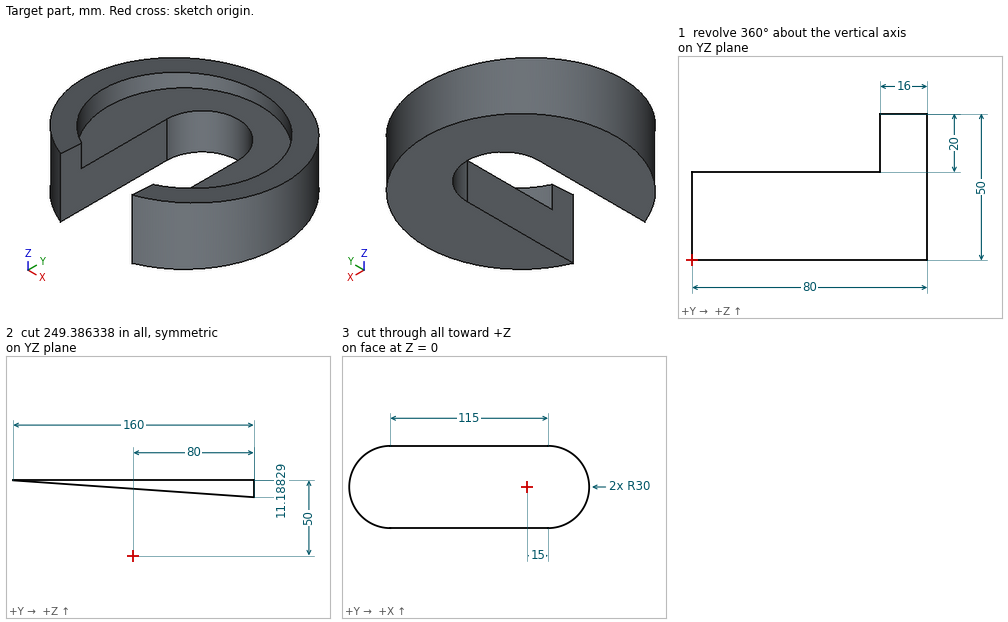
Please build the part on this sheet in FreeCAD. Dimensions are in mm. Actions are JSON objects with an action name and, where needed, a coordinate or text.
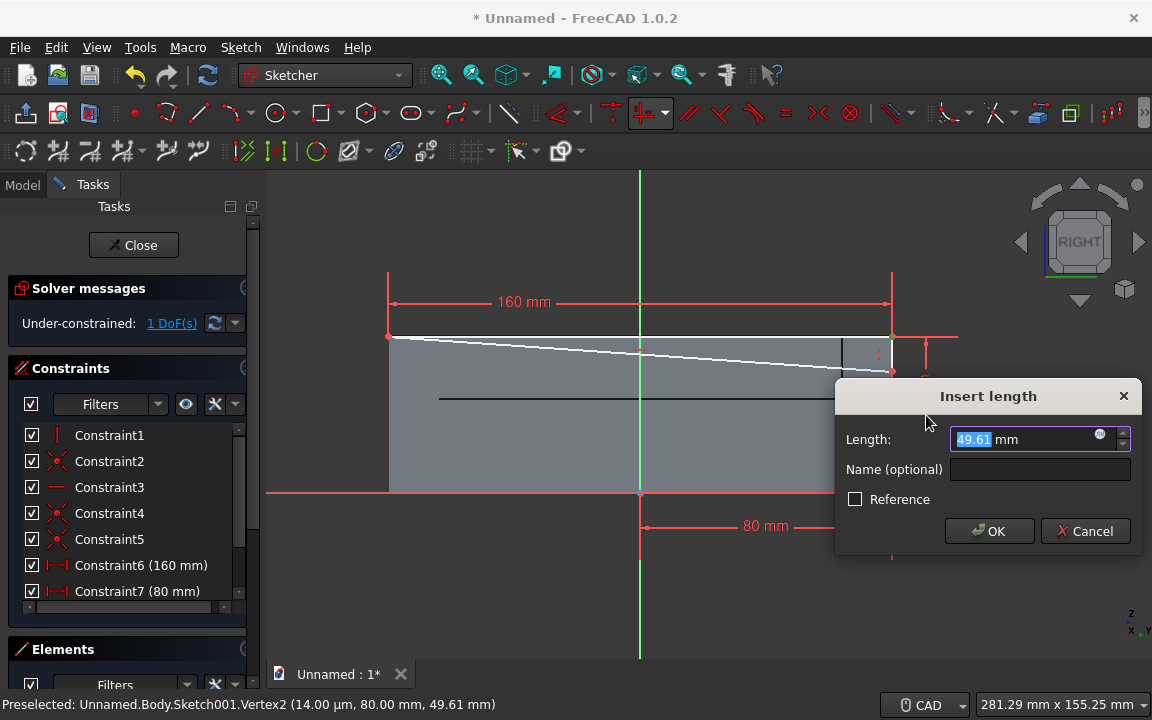
{"action": "type", "text": "50"}
{"action": "key", "text": "Return"}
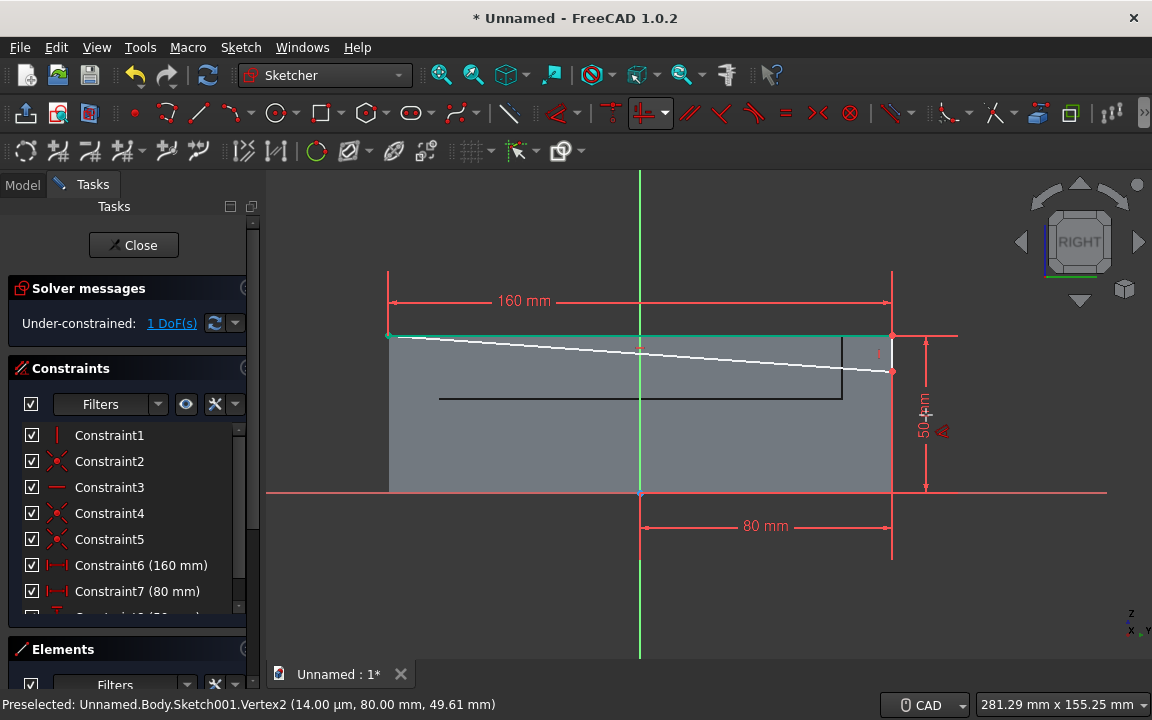
{"action": "scroll", "coordinate": [892, 361], "scroll_direction": "up", "scroll_amount": 2}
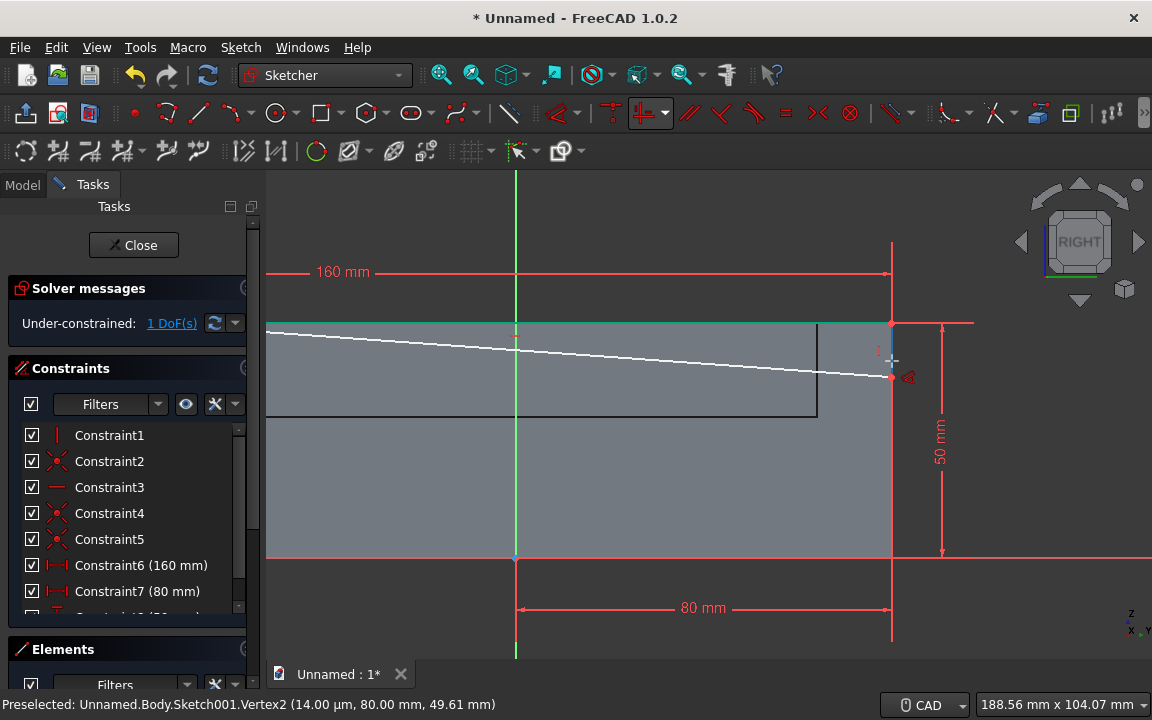
{"action": "left_click", "coordinate": [892, 361]}
{"action": "left_click", "coordinate": [926, 350]}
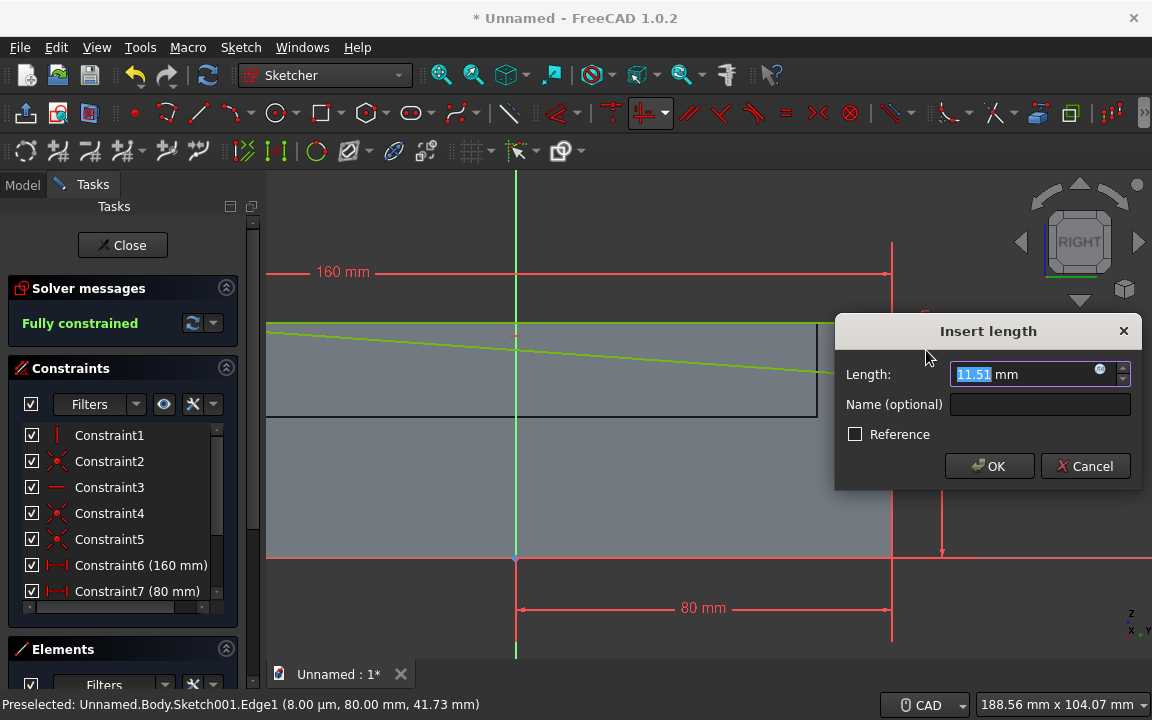
{"action": "type", "text": "11.18829"}
{"action": "key", "text": "Return"}
{"action": "key", "text": "Escape"}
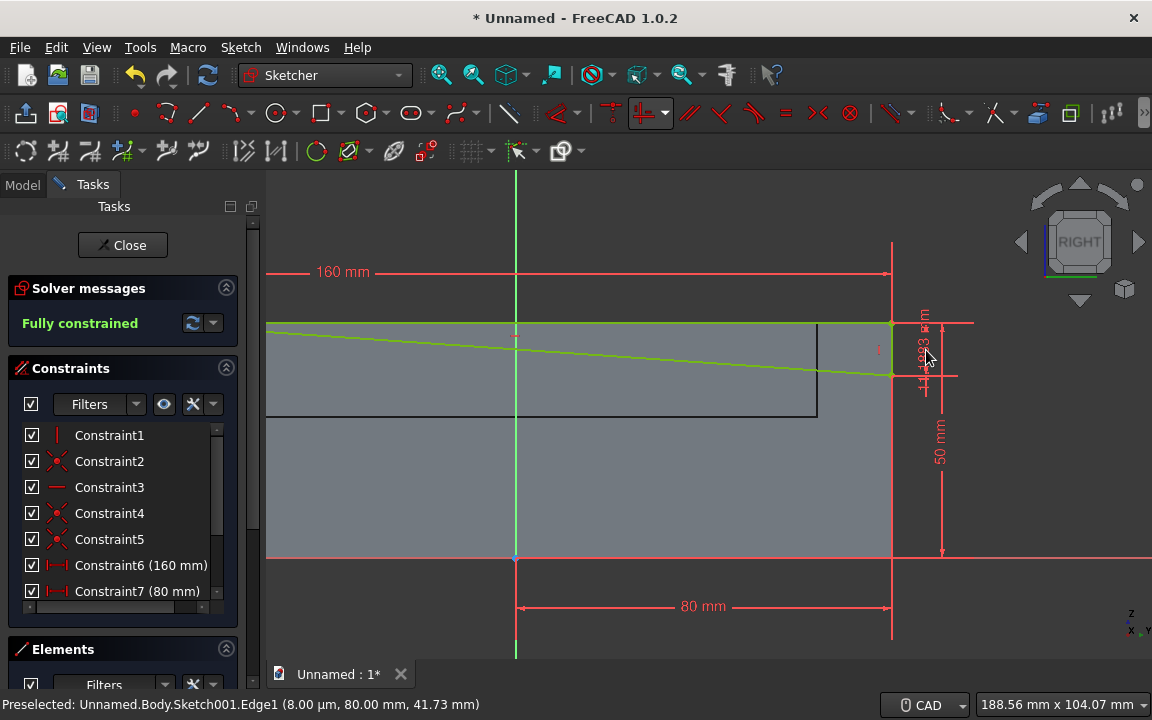
{"action": "left_click", "coordinate": [123, 245]}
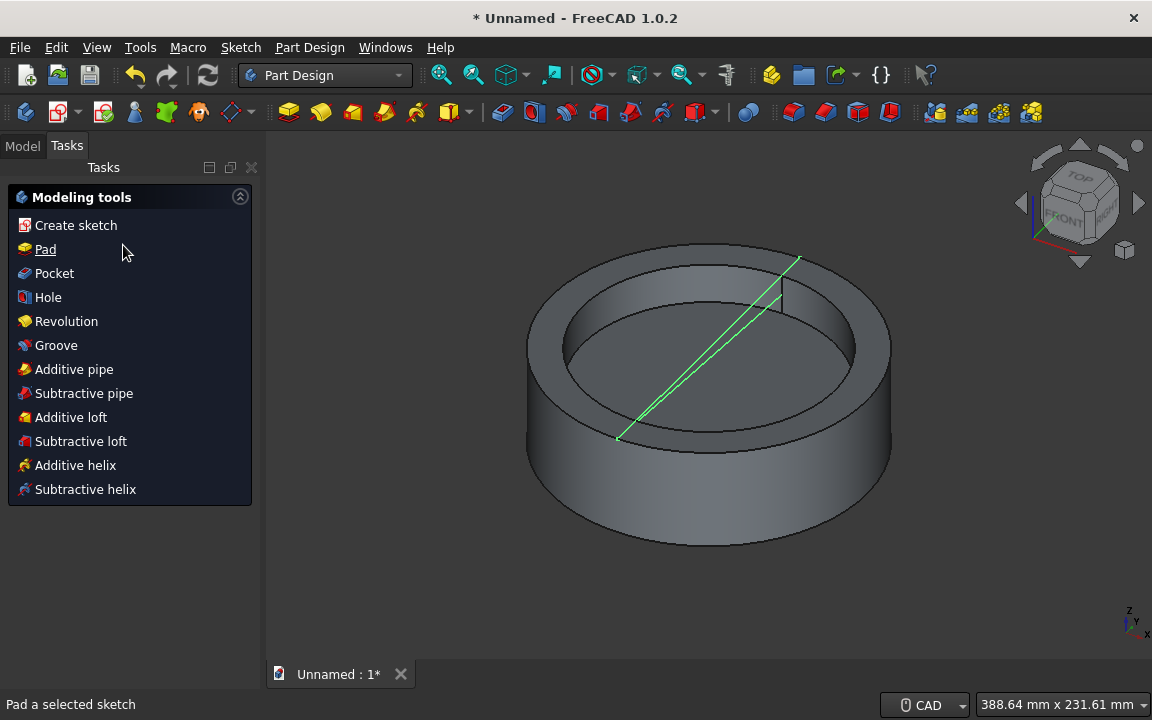
{"action": "left_click", "coordinate": [504, 112]}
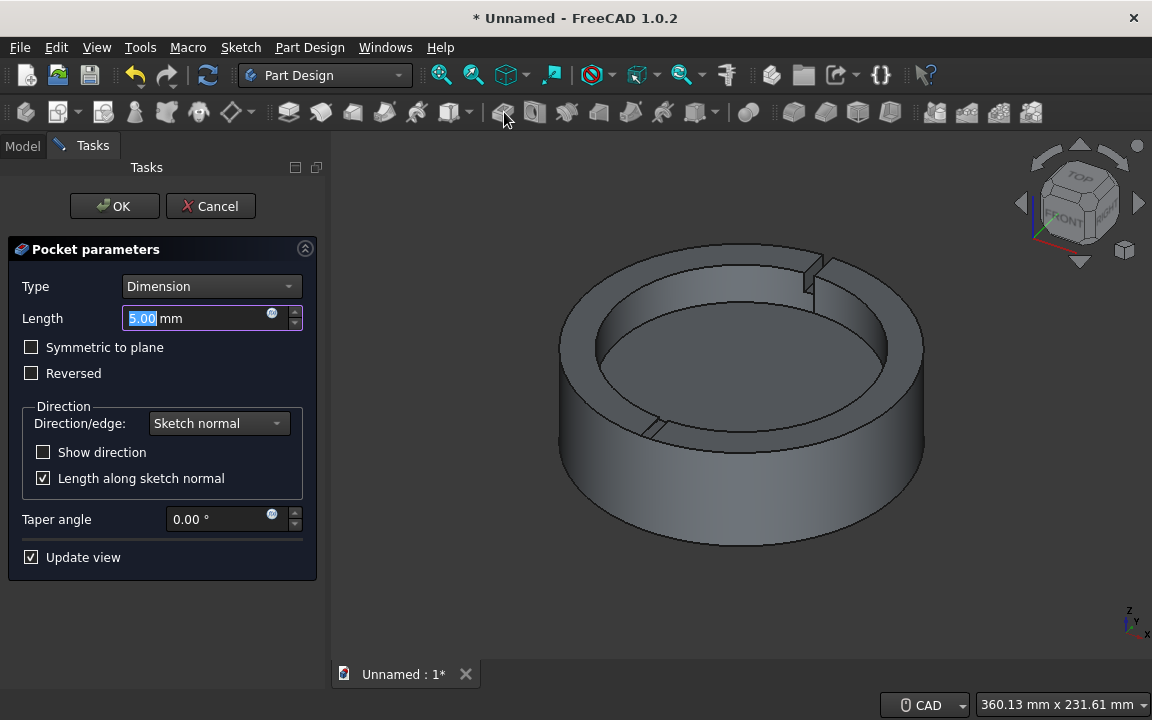
{"action": "type", "text": "249.386338"}
{"action": "key", "text": "Tab"}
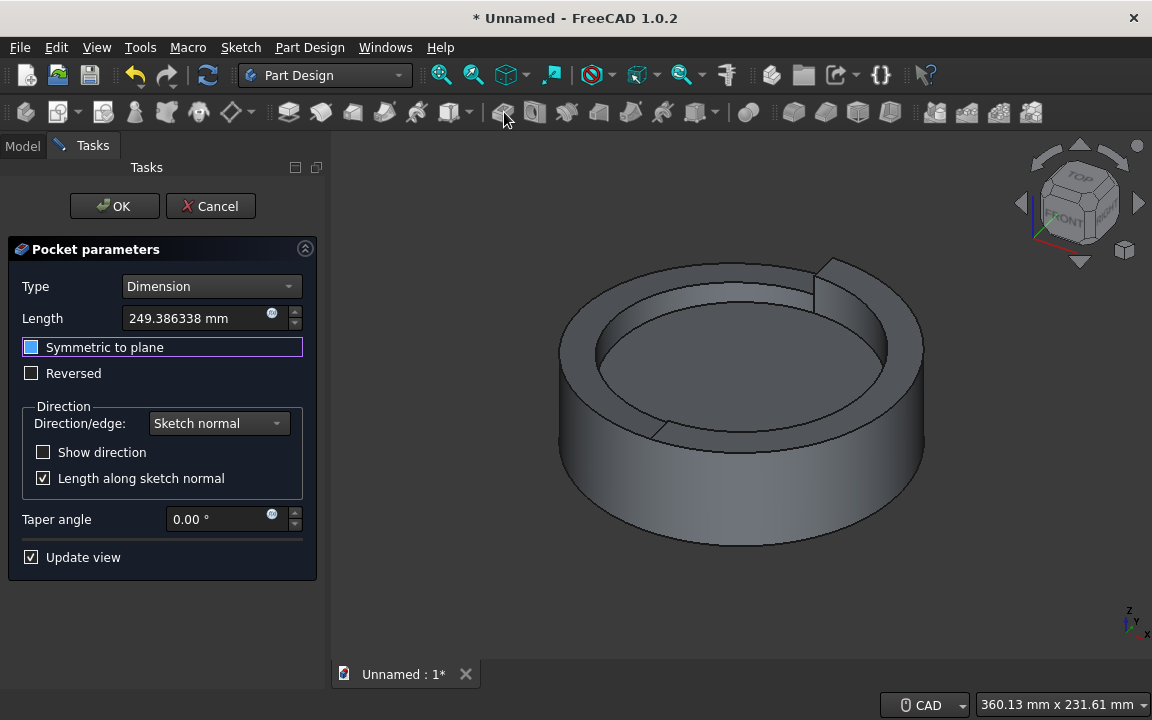
{"action": "left_click", "coordinate": [30, 347]}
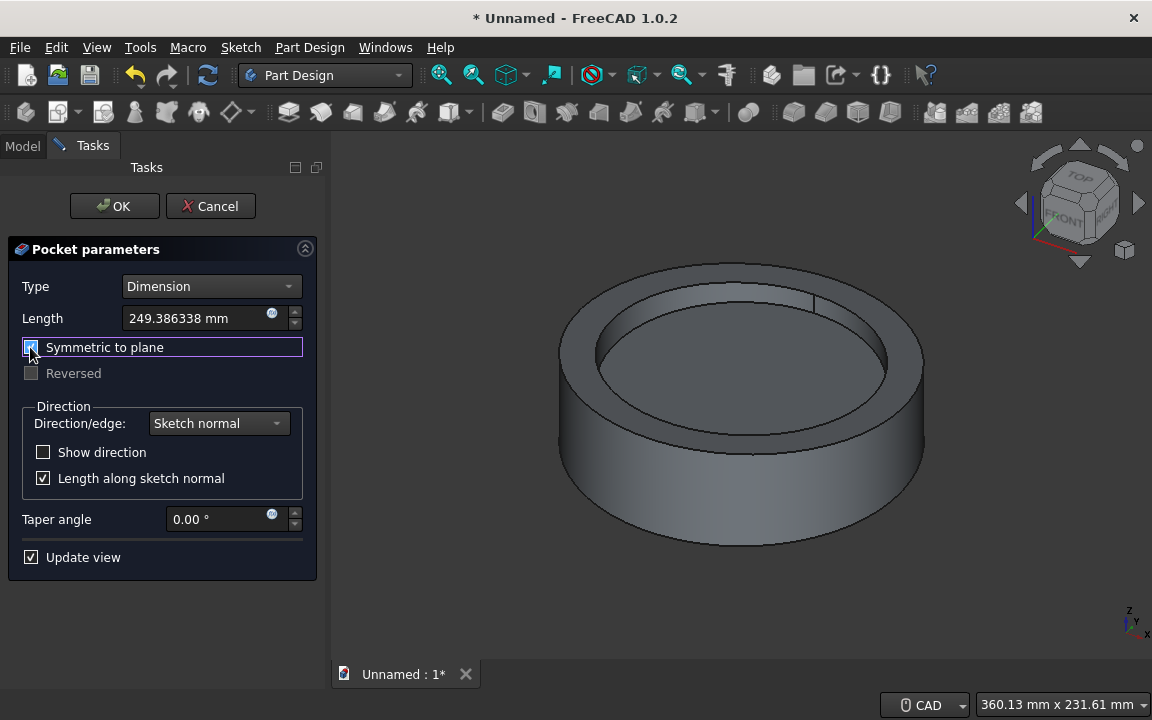
{"action": "left_click", "coordinate": [115, 206]}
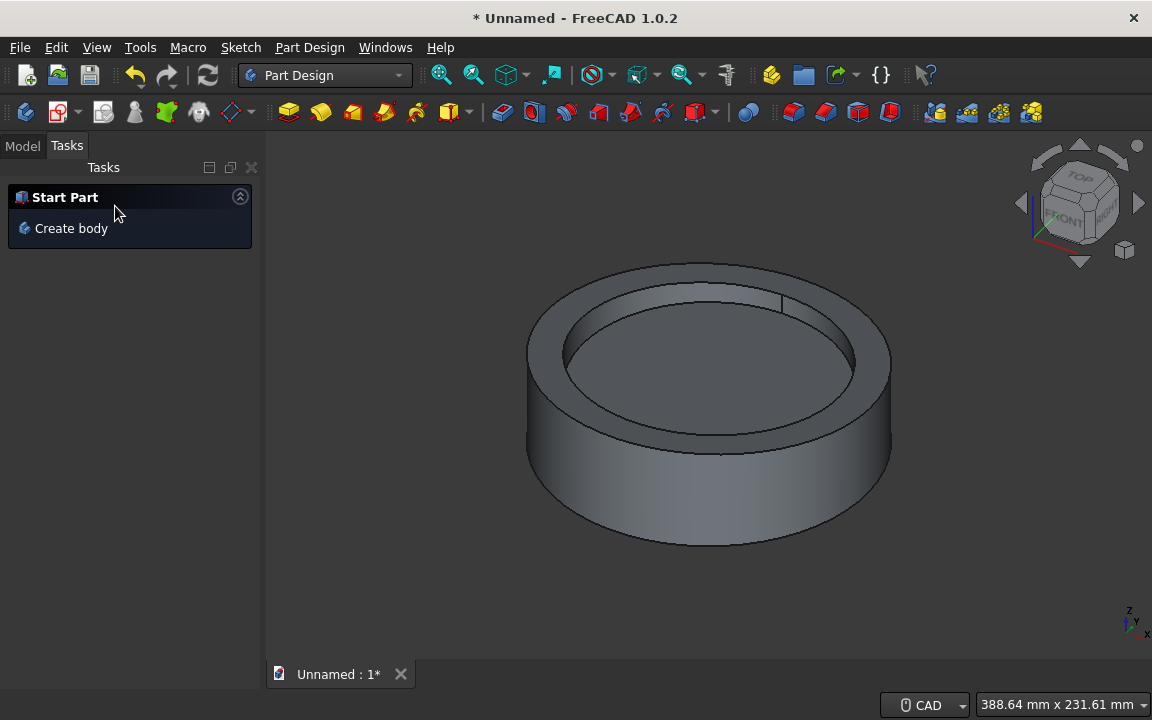
{"action": "key", "text": "5"}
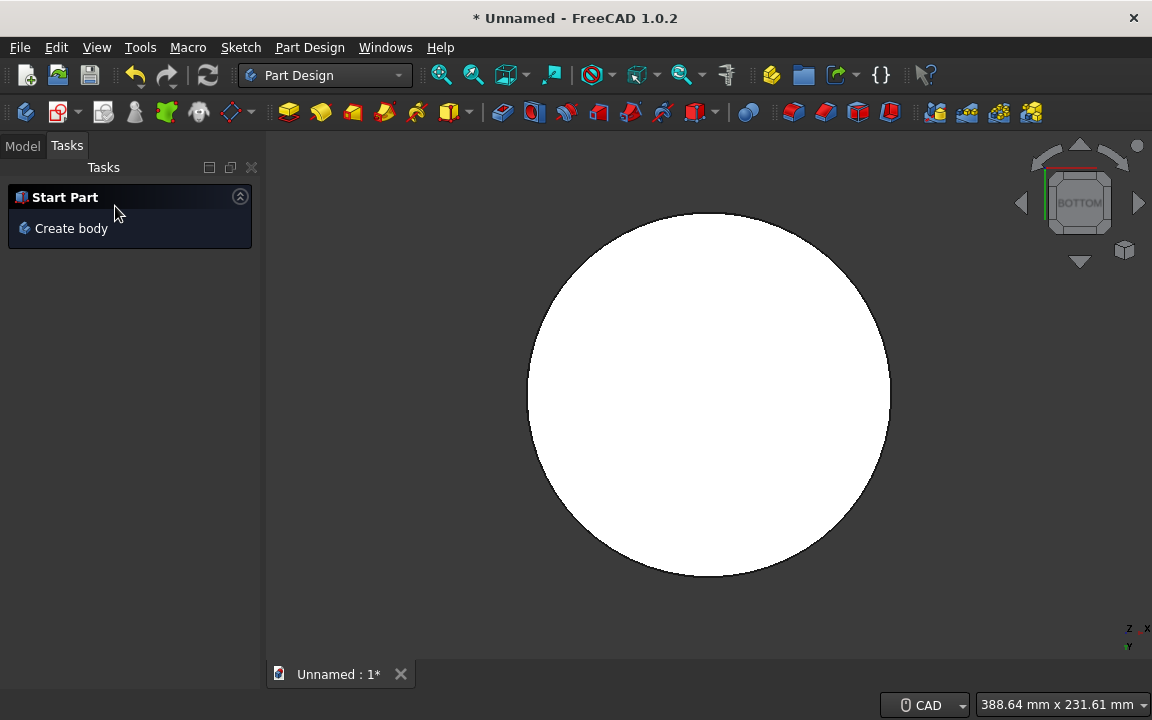
{"action": "left_click", "coordinate": [709, 394]}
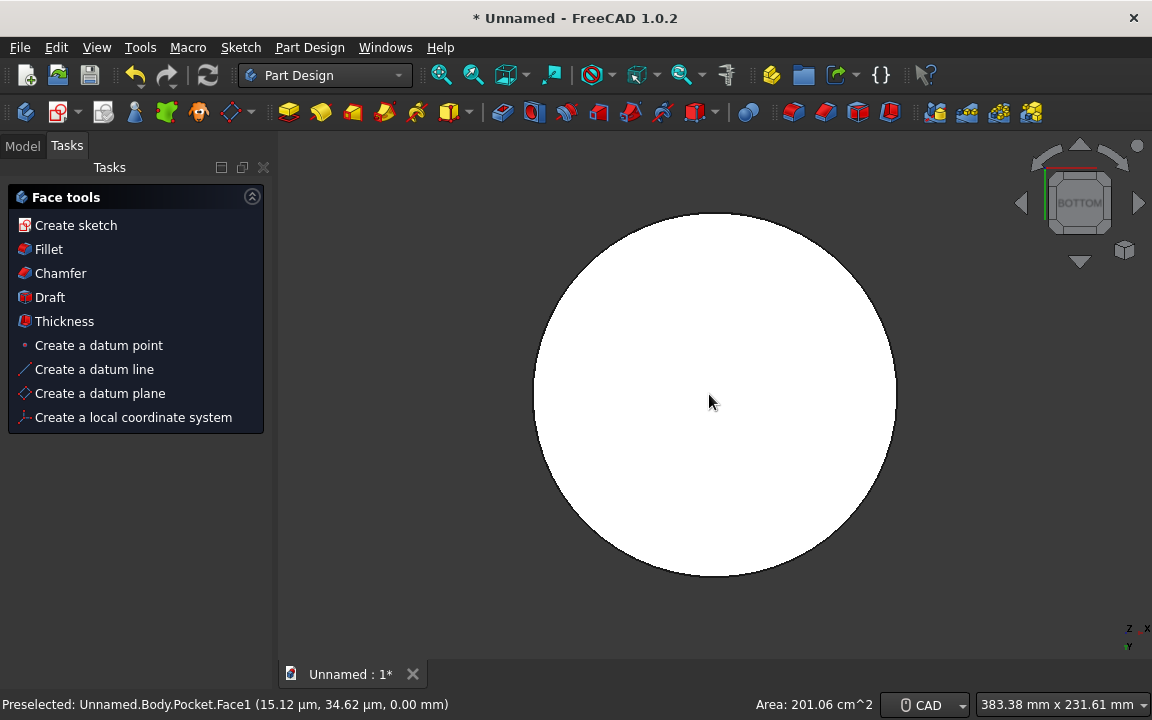
{"action": "left_click", "coordinate": [58, 112]}